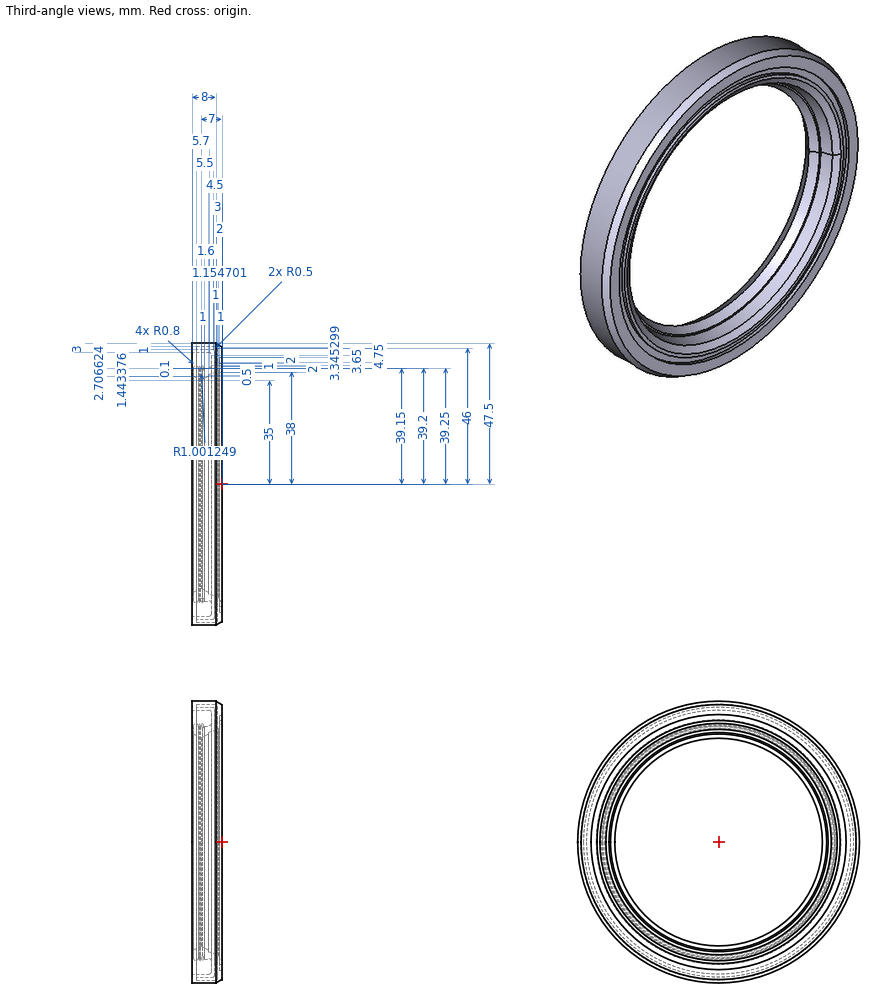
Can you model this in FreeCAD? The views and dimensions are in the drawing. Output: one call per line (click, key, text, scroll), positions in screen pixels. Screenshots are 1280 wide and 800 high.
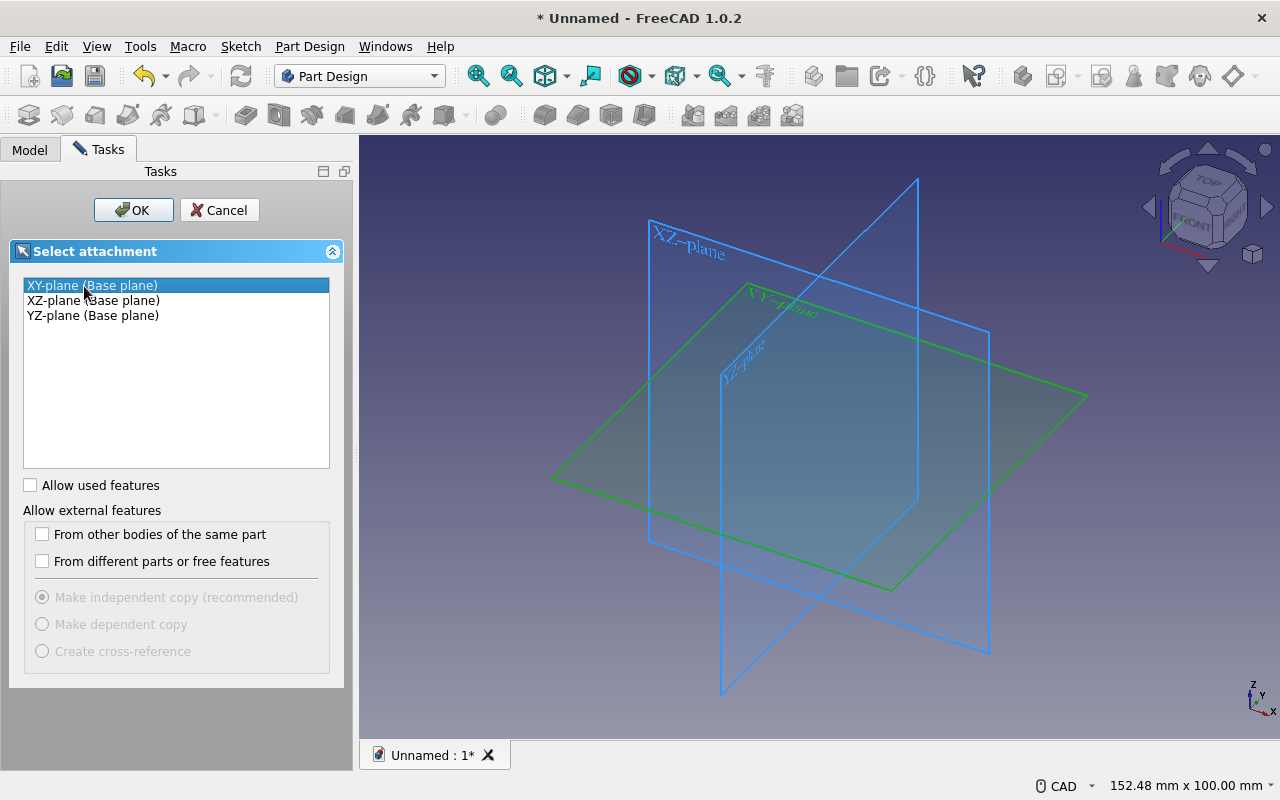
click(134, 210)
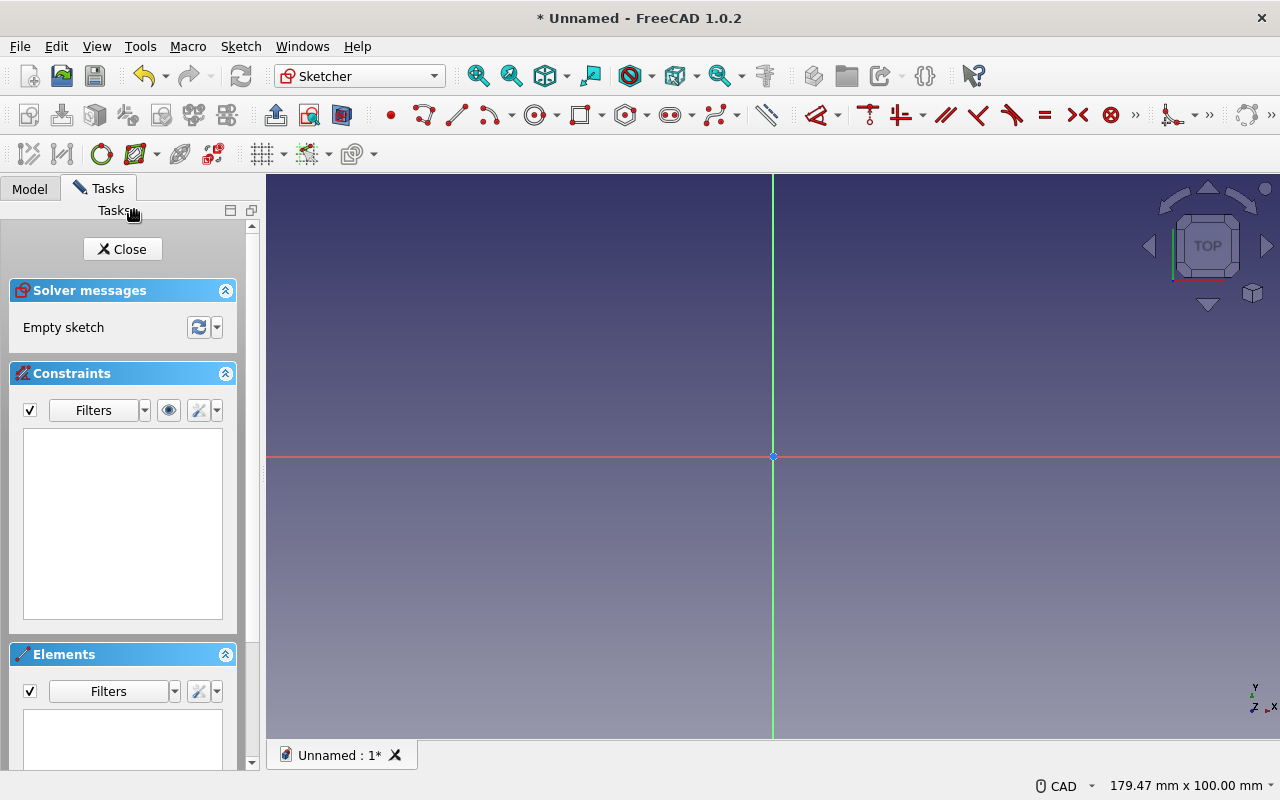
scroll(704, 456, down, 5)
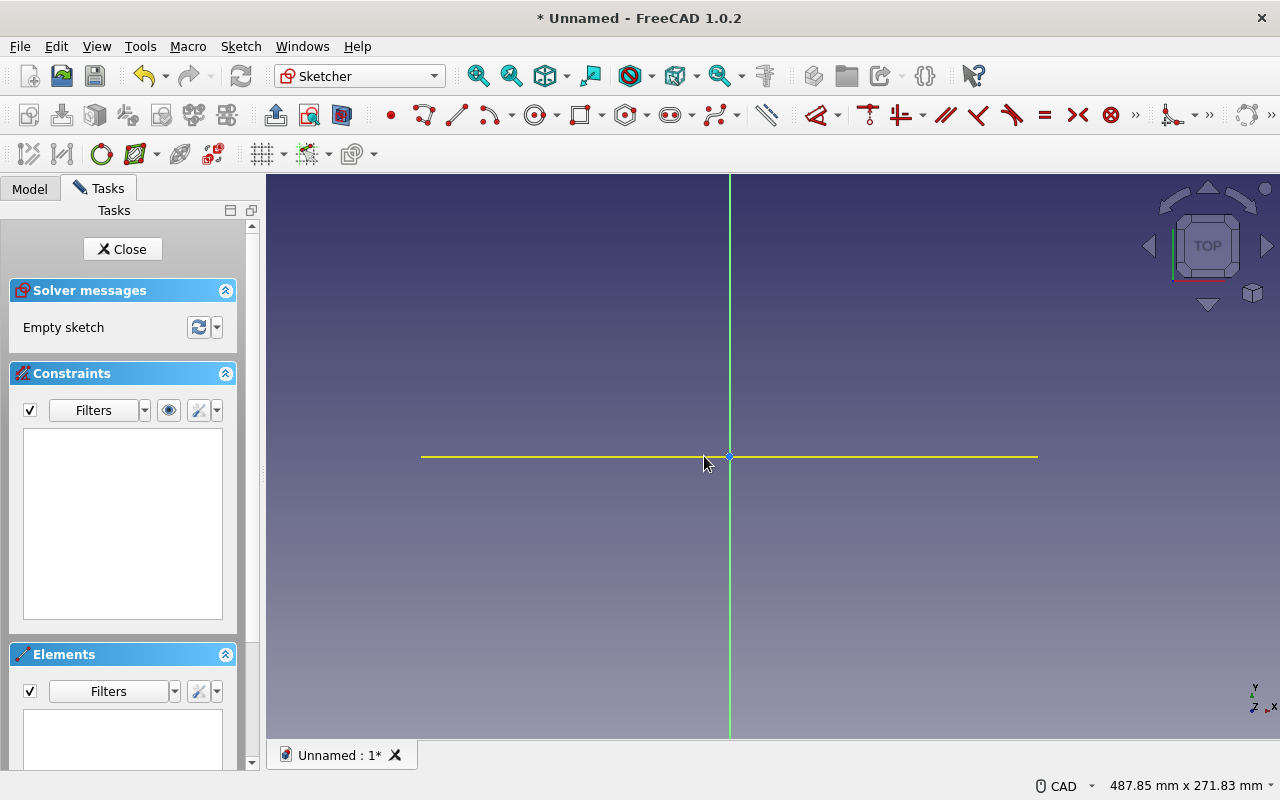
scroll(720, 364, up, 13)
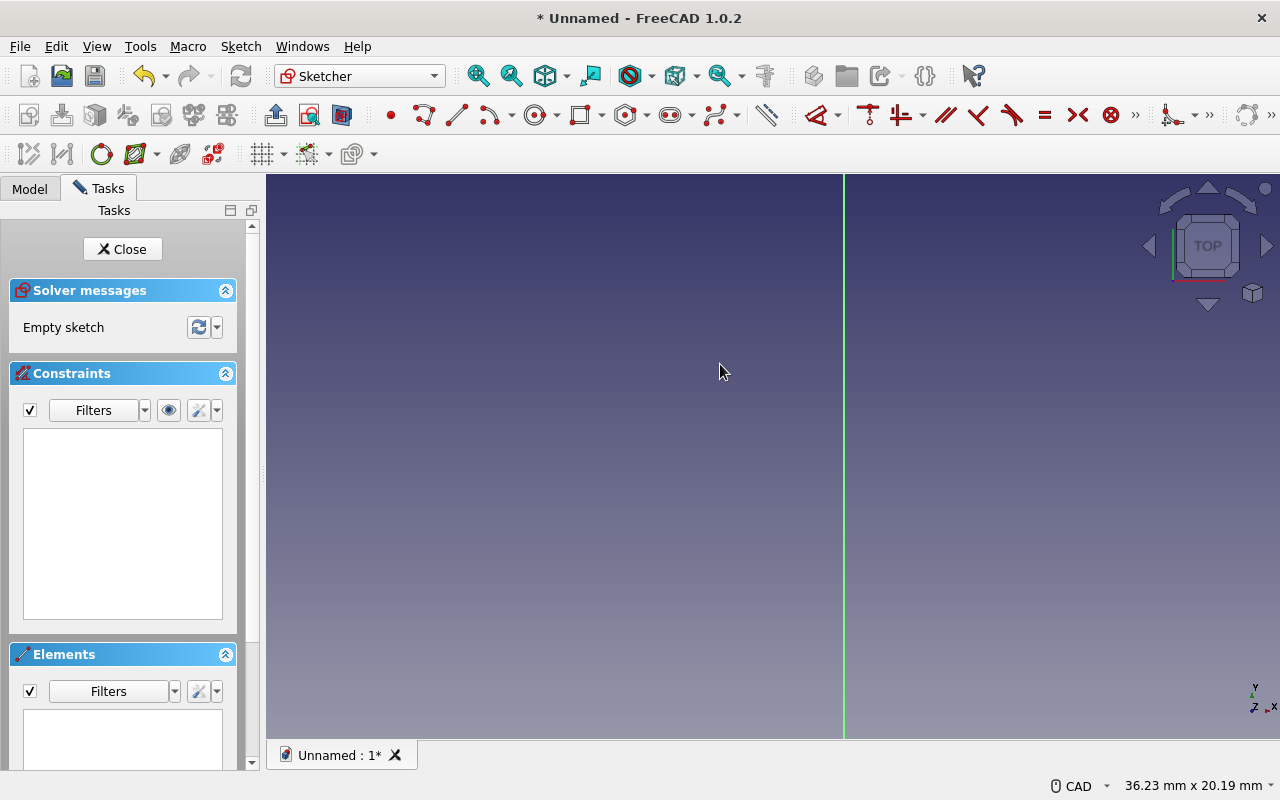
click(424, 116)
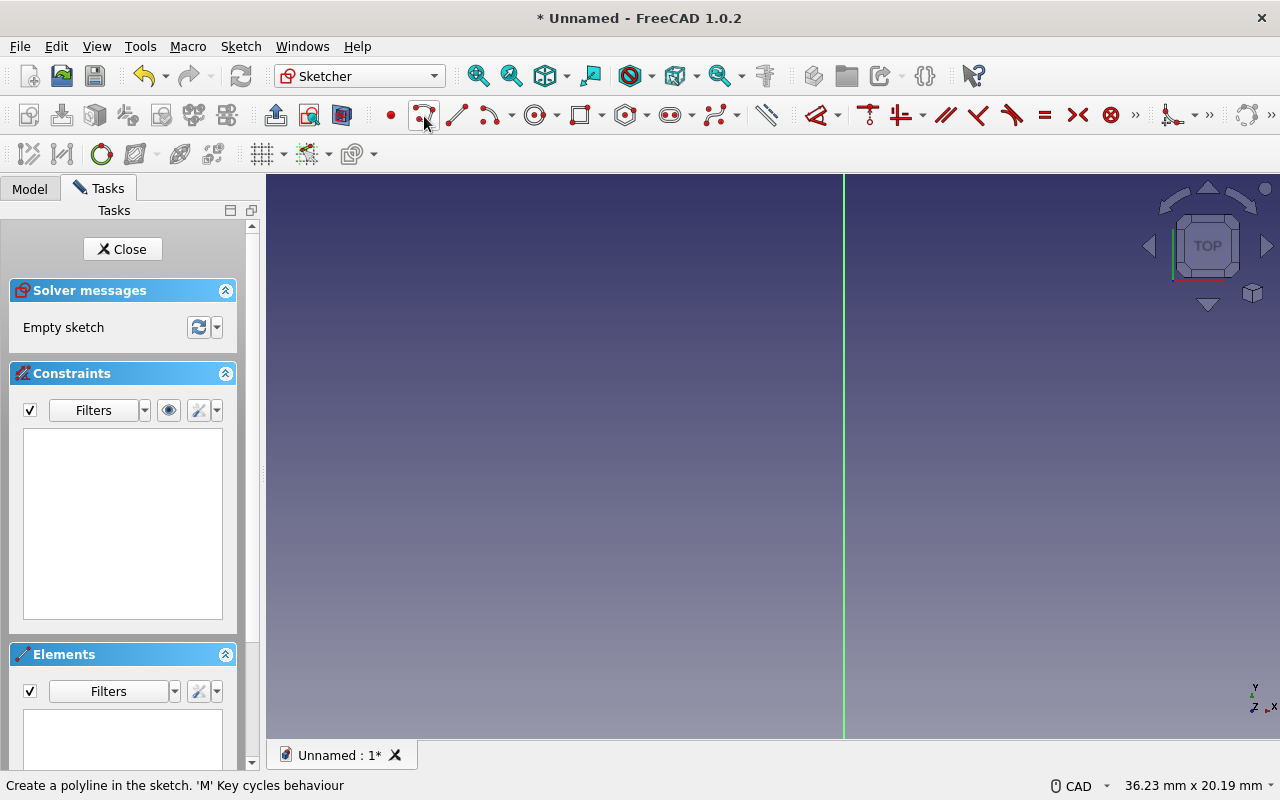
click(579, 510)
click(579, 585)
click(649, 626)
click(719, 585)
click(719, 571)
click(812, 542)
click(844, 486)
click(835, 458)
click(816, 458)
click(816, 402)
click(844, 402)
click(835, 308)
click(788, 276)
click(565, 276)
click(565, 360)
click(724, 360)
right_click(724, 360)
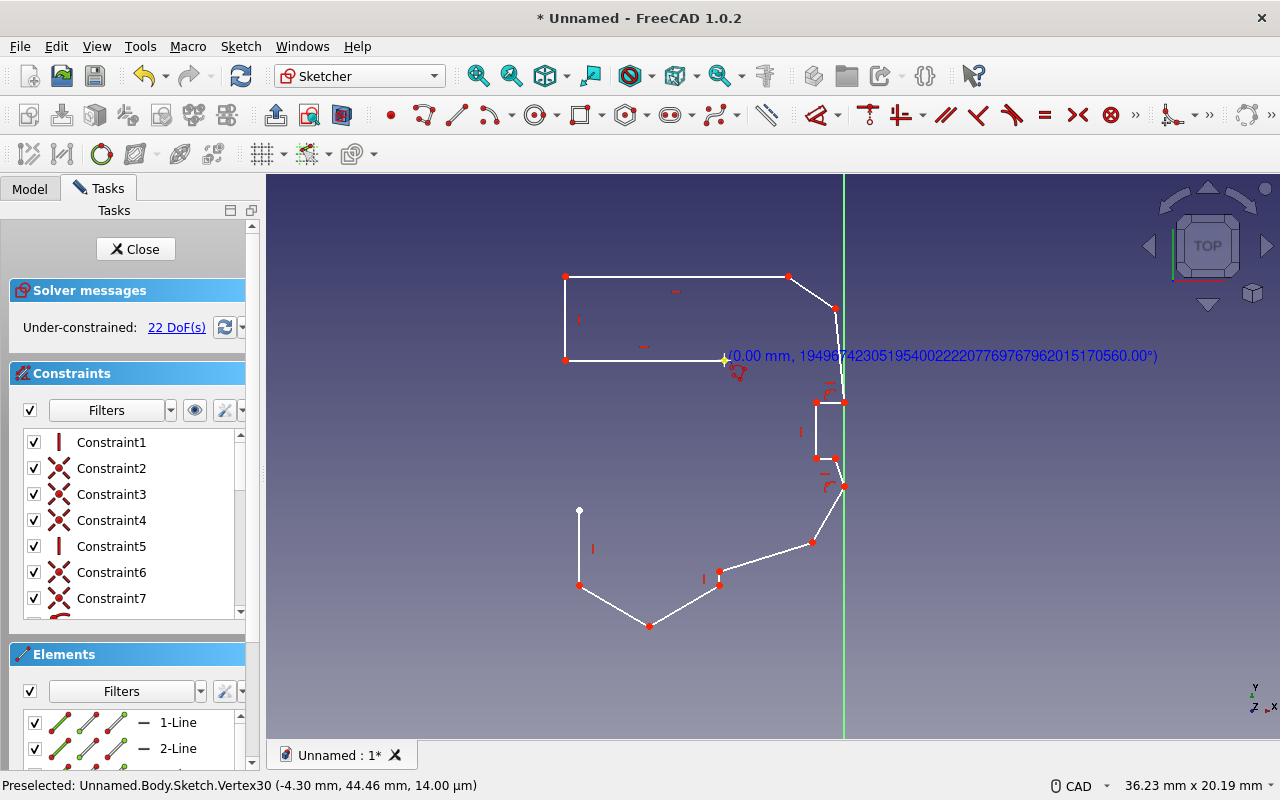
key(g)
key(l)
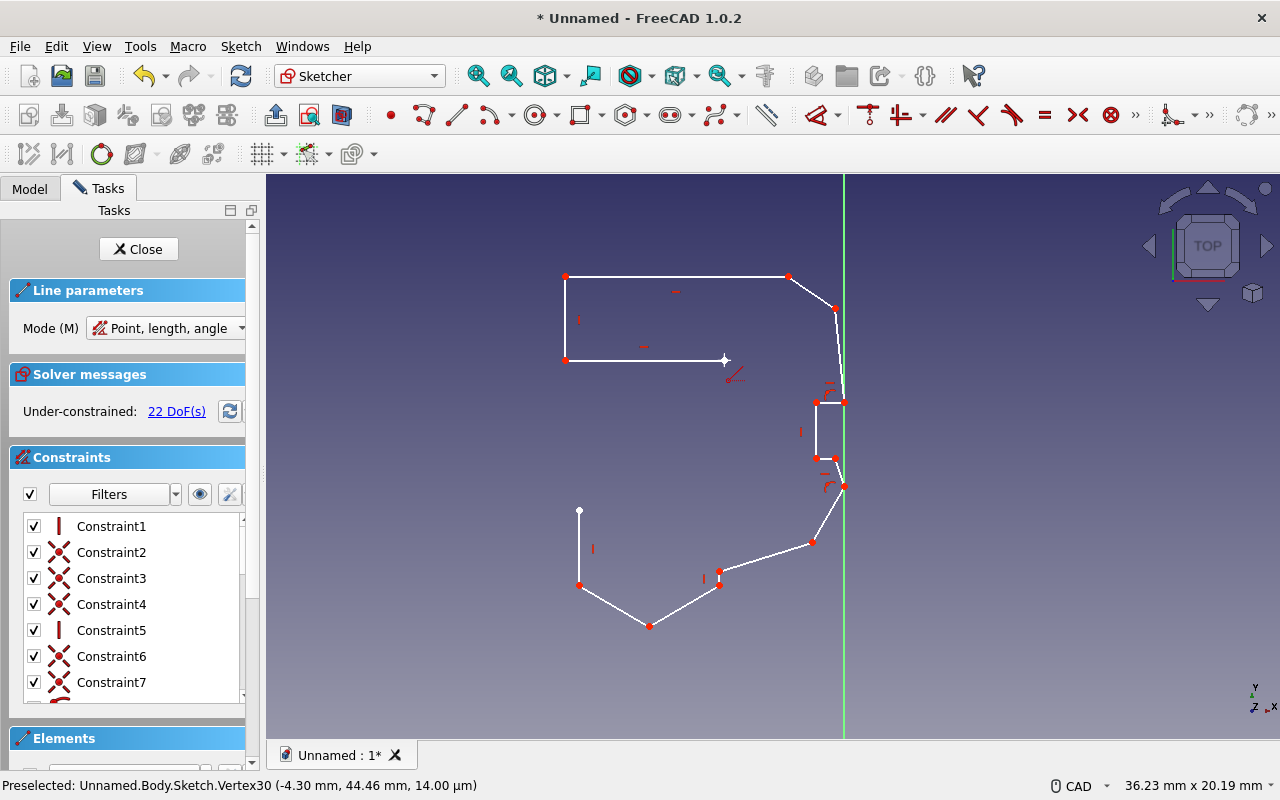
click(746, 382)
click(746, 484)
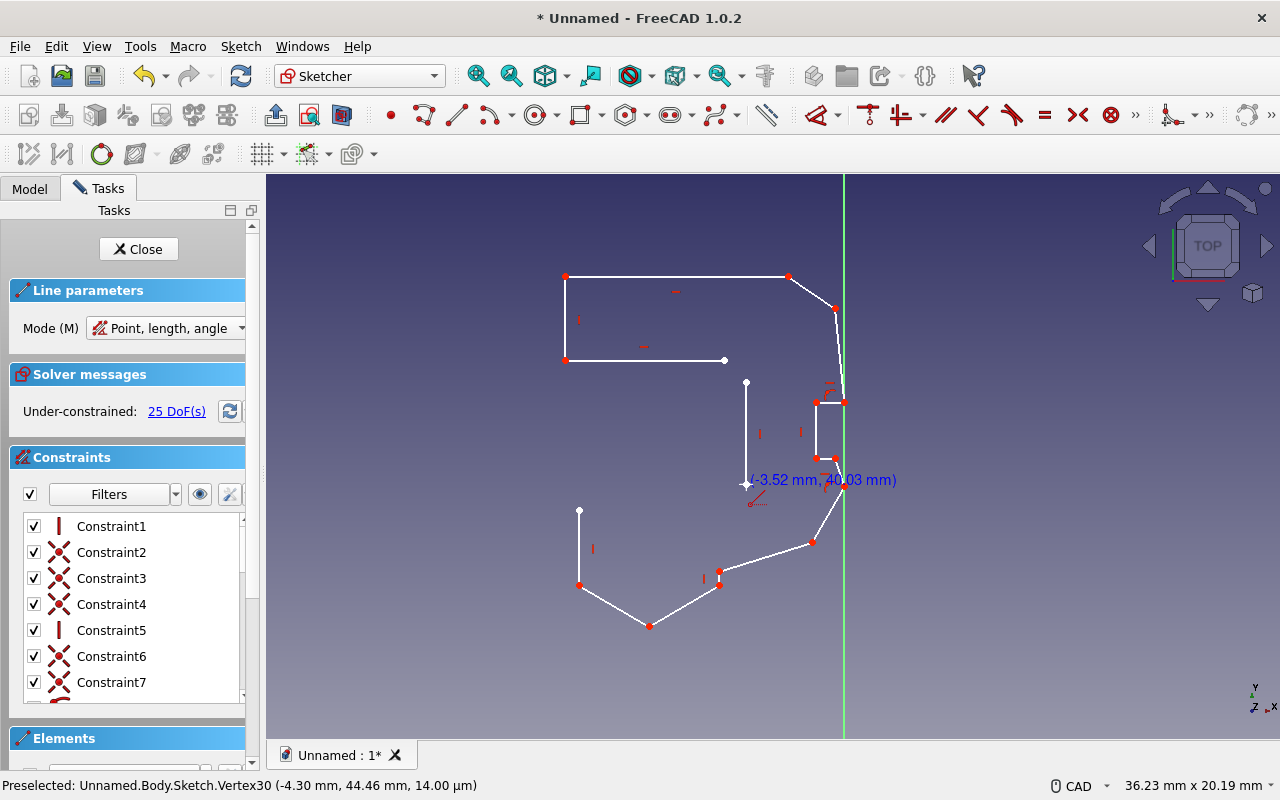
click(724, 507)
click(679, 507)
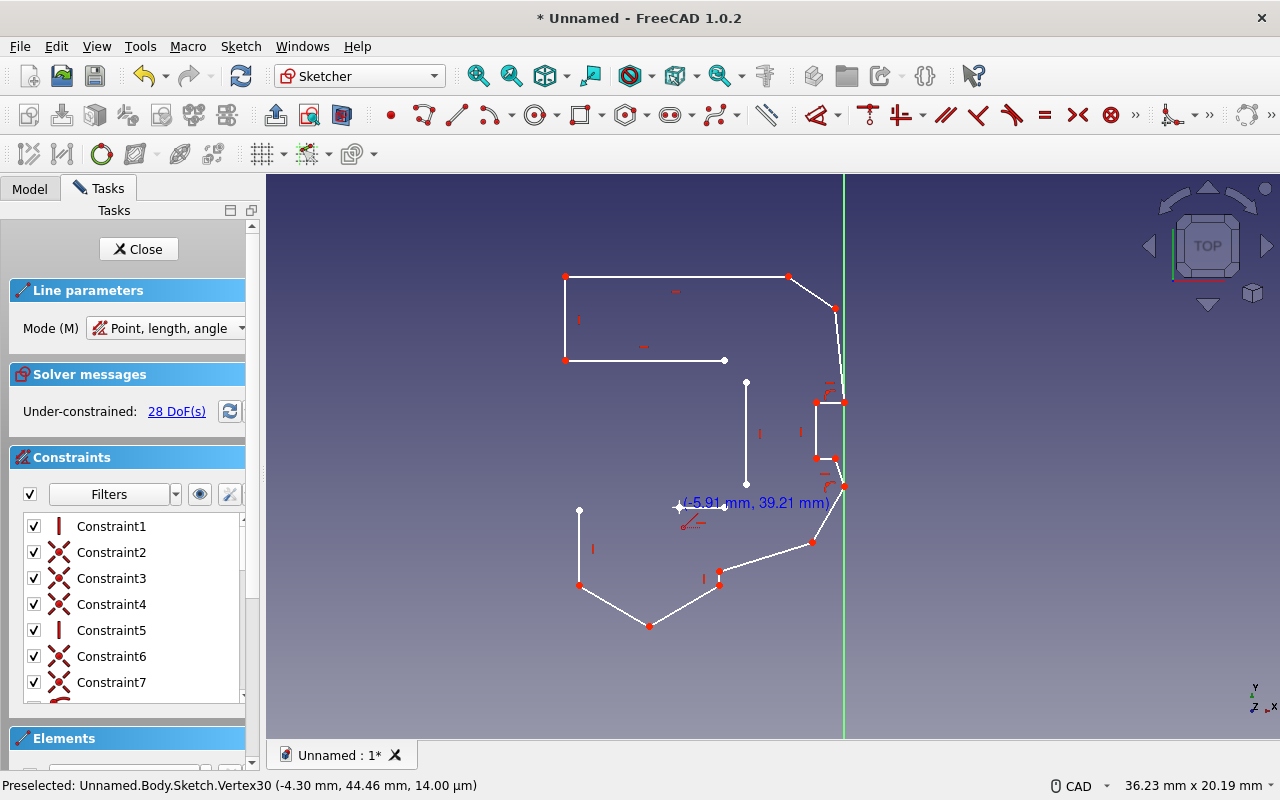
key(g)
key(3)
key(a)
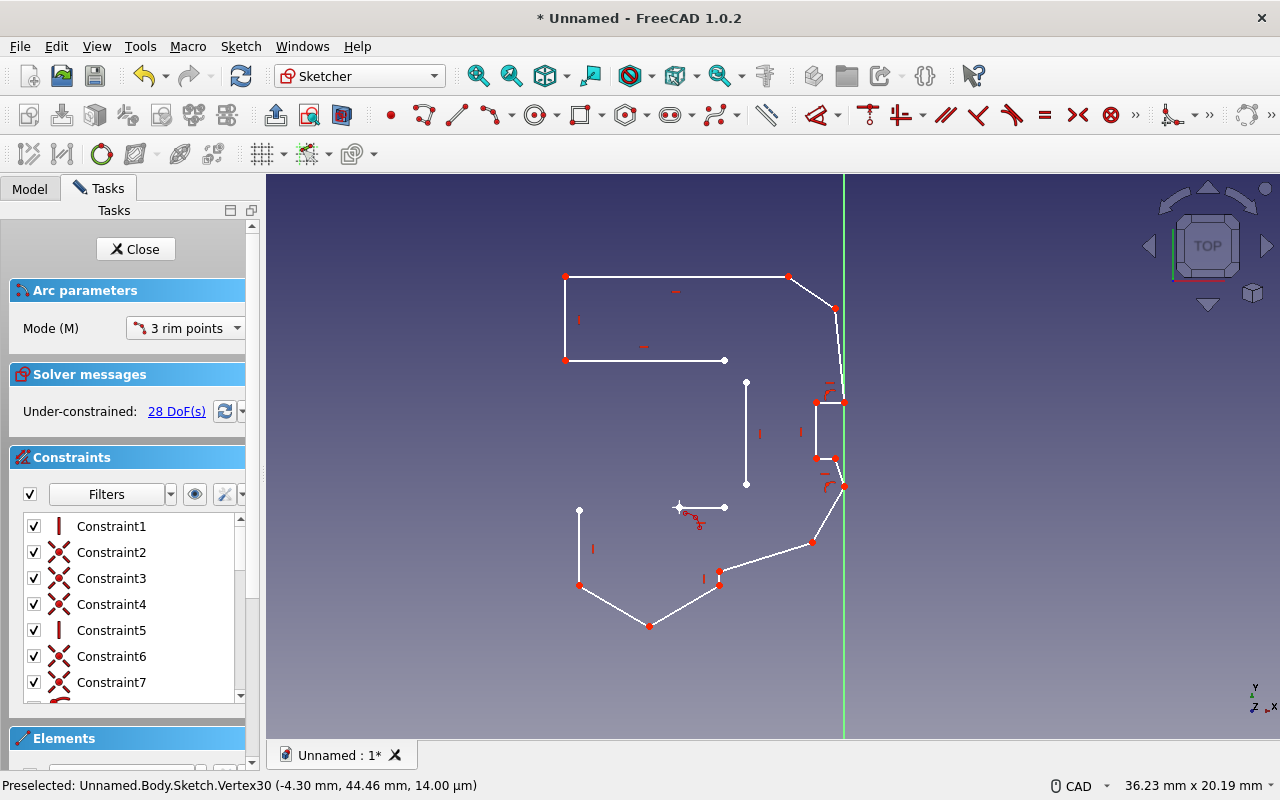
click(724, 361)
click(746, 383)